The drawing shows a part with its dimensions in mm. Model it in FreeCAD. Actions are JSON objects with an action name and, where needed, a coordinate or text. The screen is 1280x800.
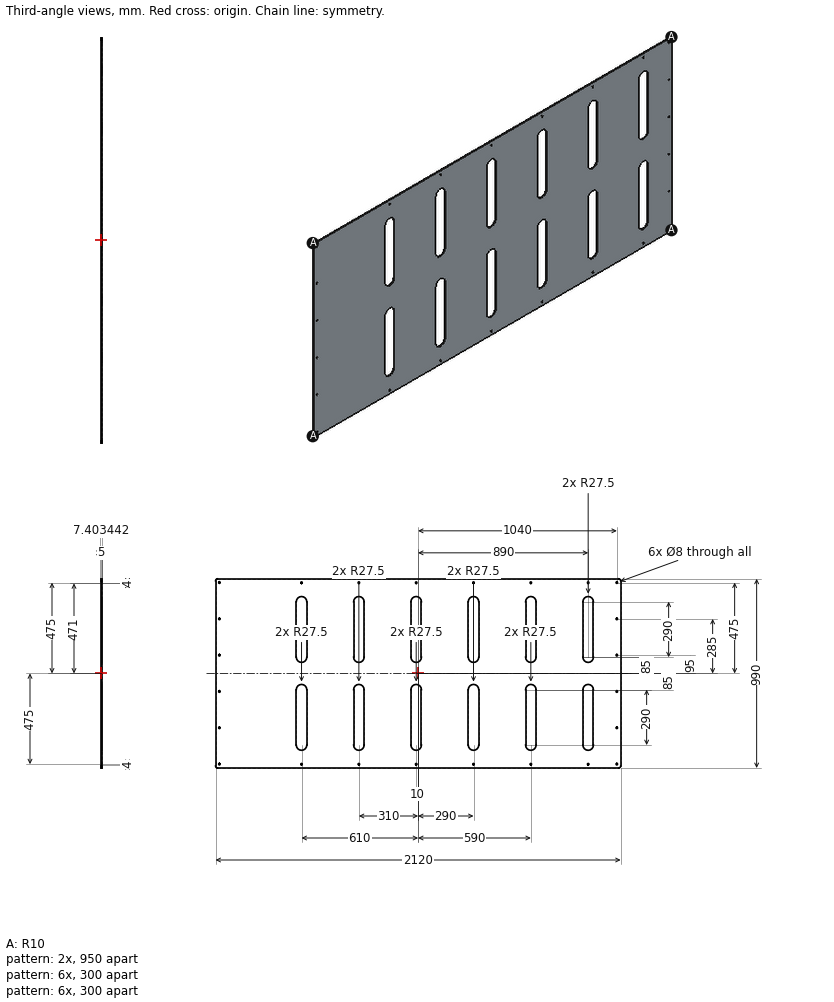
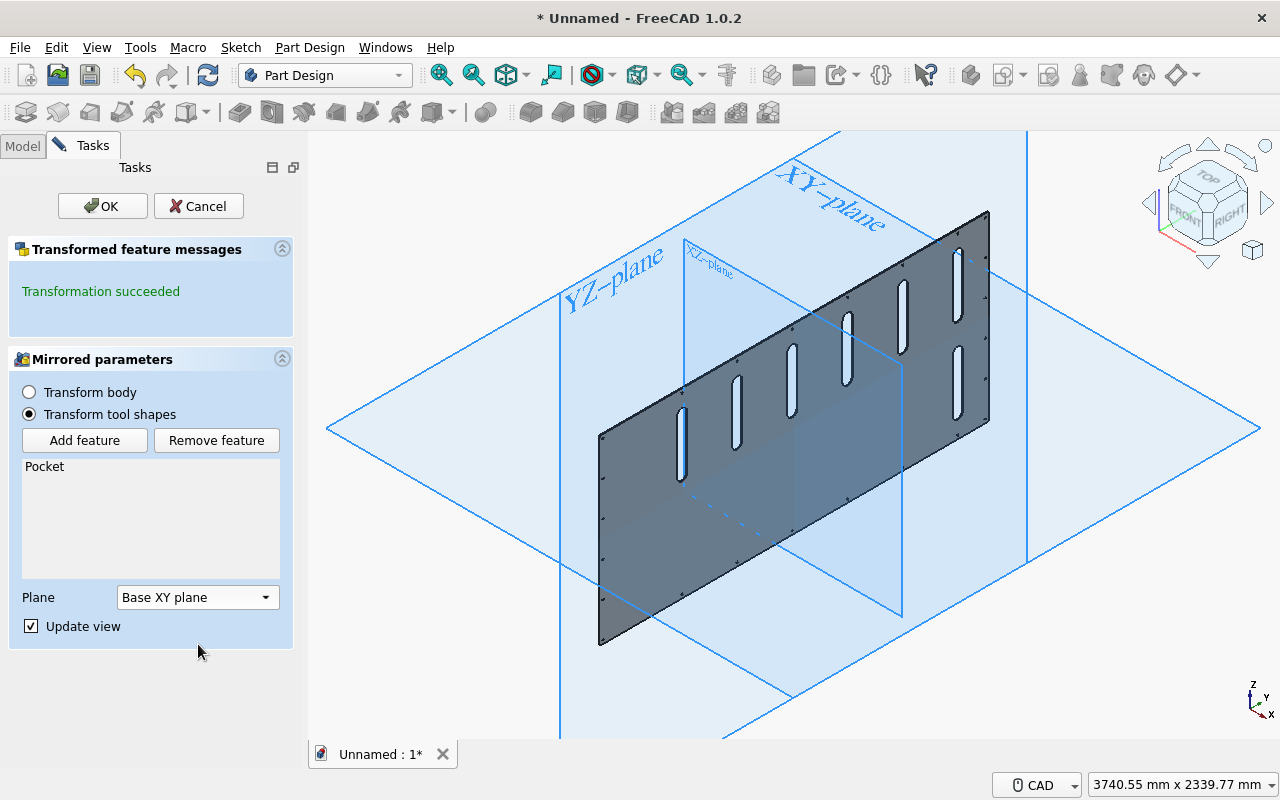
{"action": "left_click", "coordinate": [103, 206]}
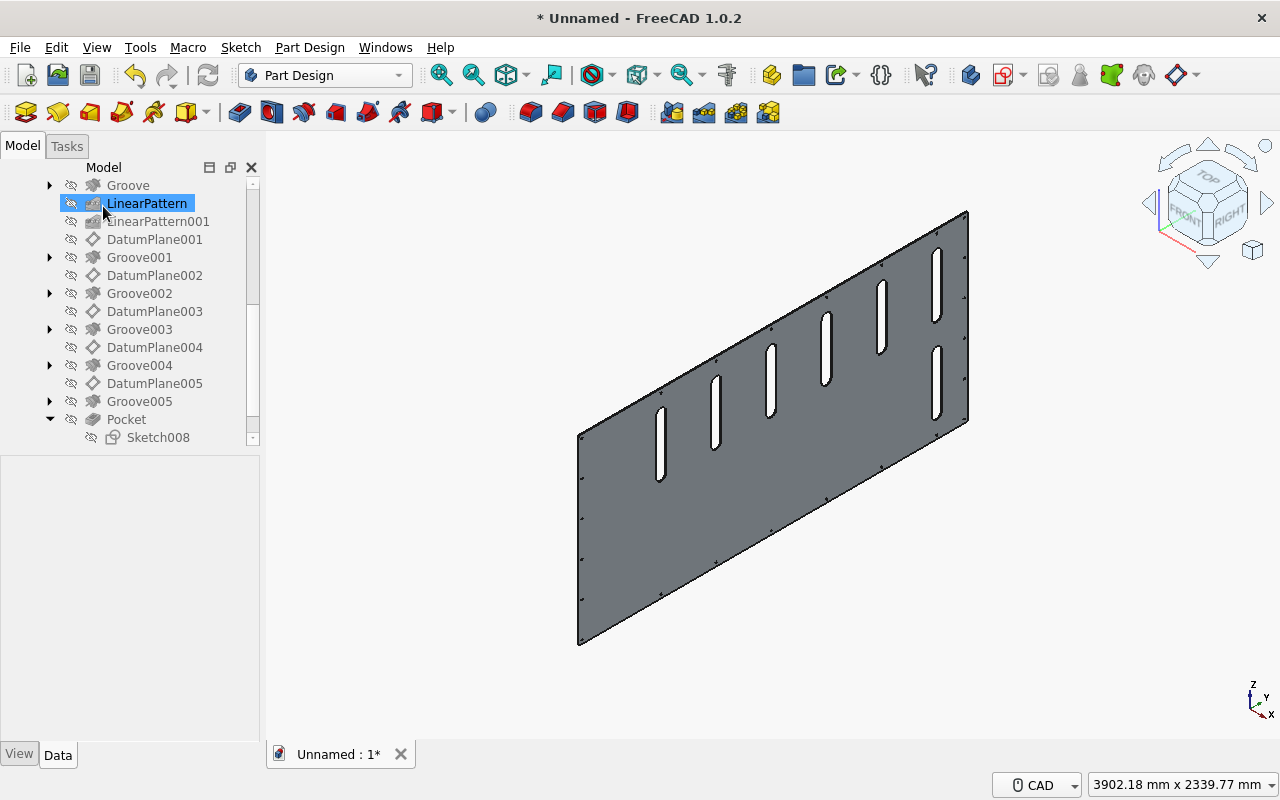
{"action": "left_click", "coordinate": [885, 393]}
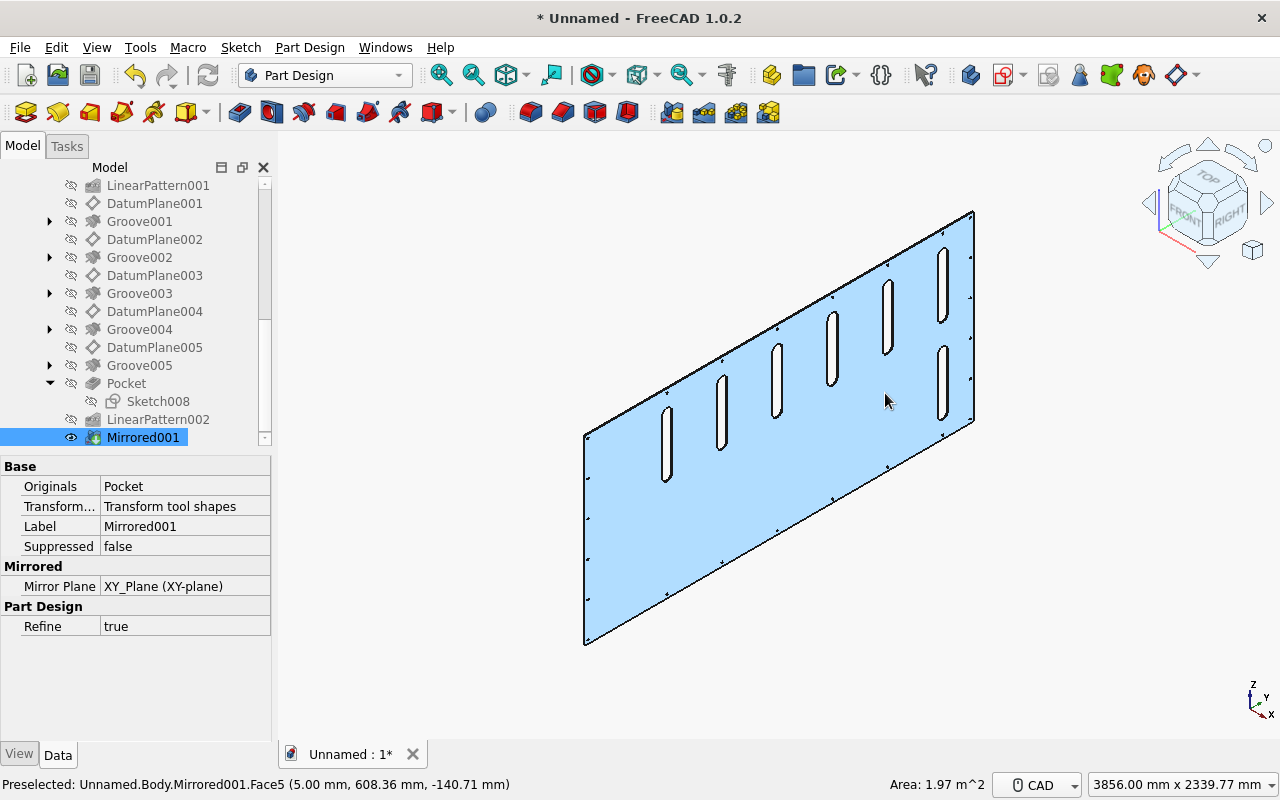
{"action": "left_click", "coordinate": [1004, 76]}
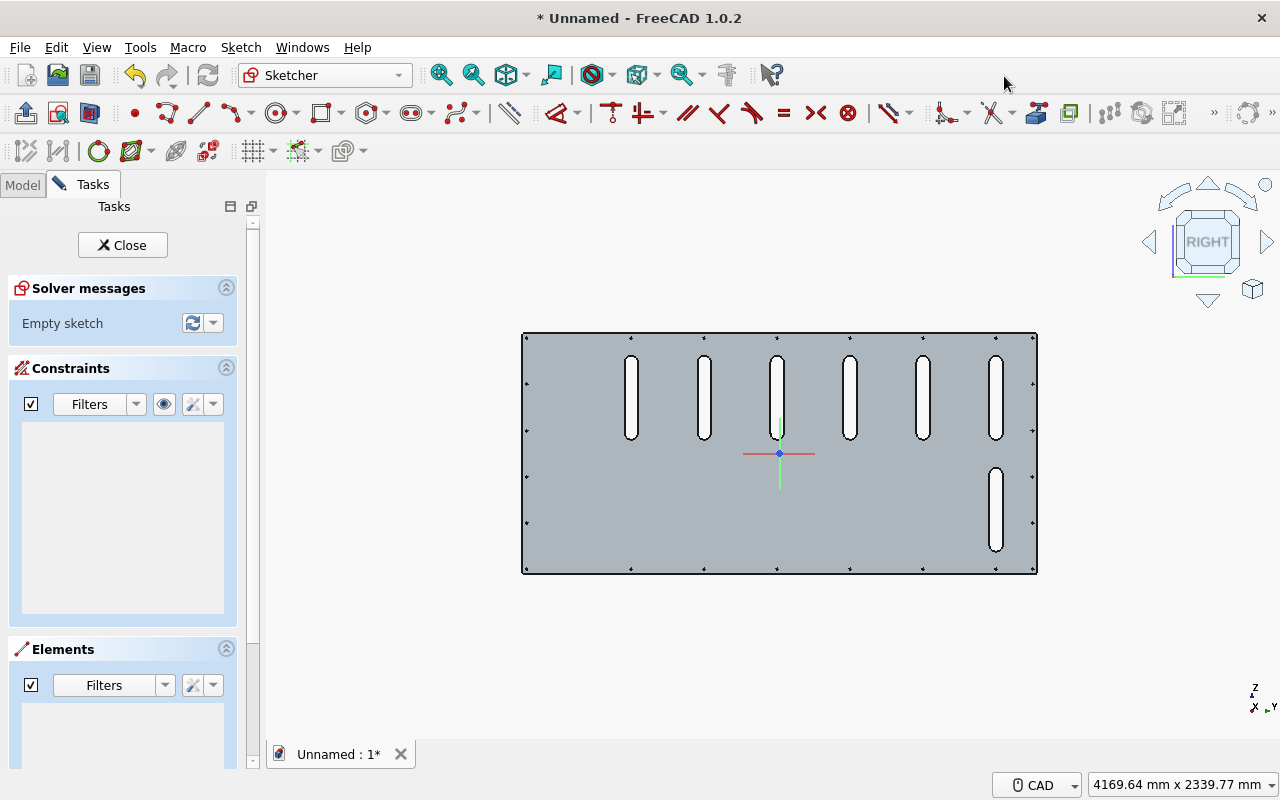
{"action": "scroll", "coordinate": [904, 518], "scroll_direction": "up", "scroll_amount": 7}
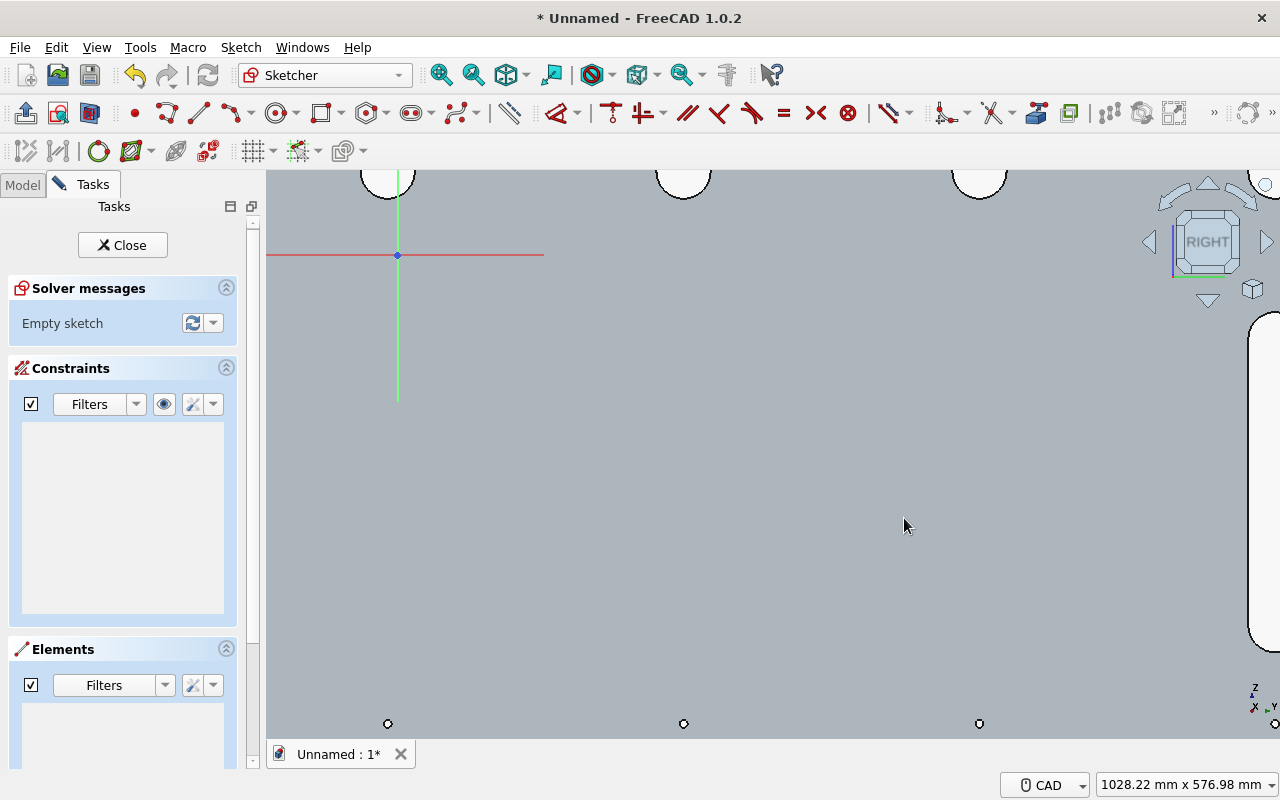
{"action": "left_click", "coordinate": [412, 114]}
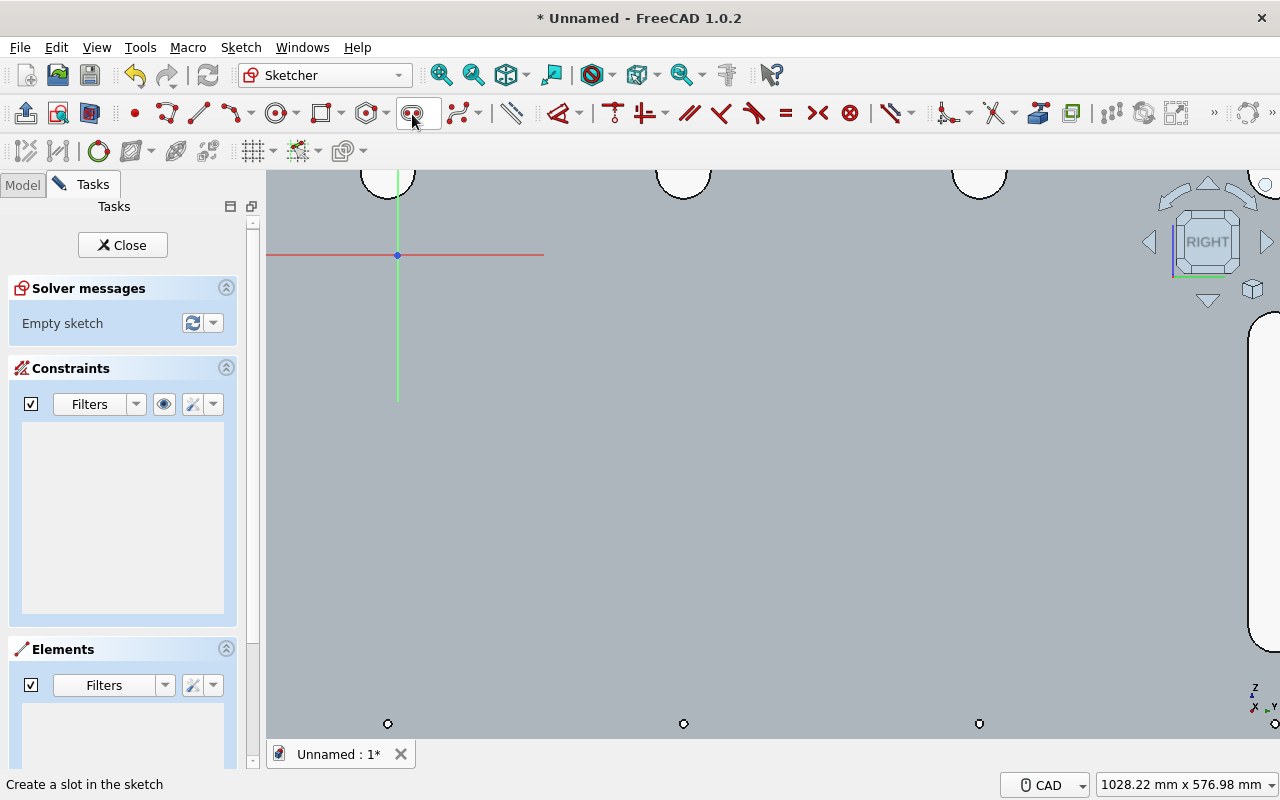
{"action": "left_click", "coordinate": [979, 625]}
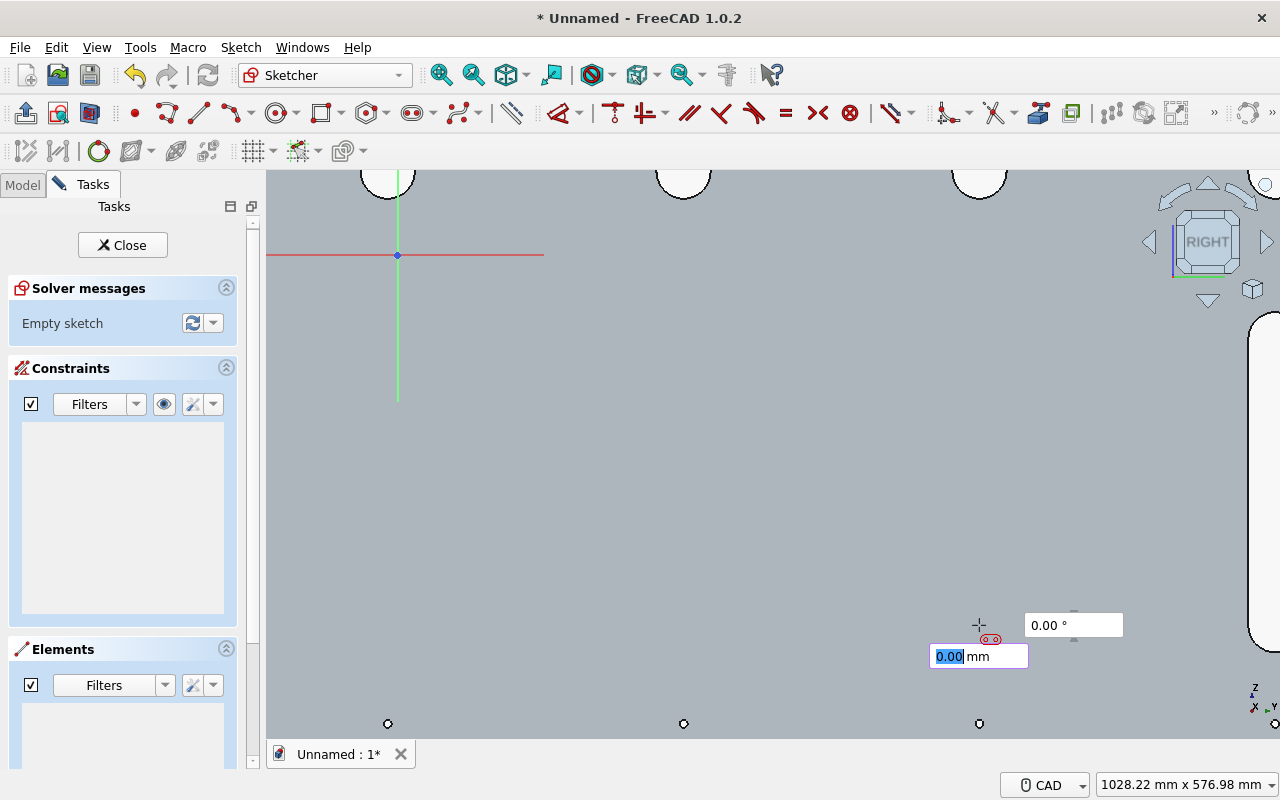
{"action": "left_click", "coordinate": [979, 339]}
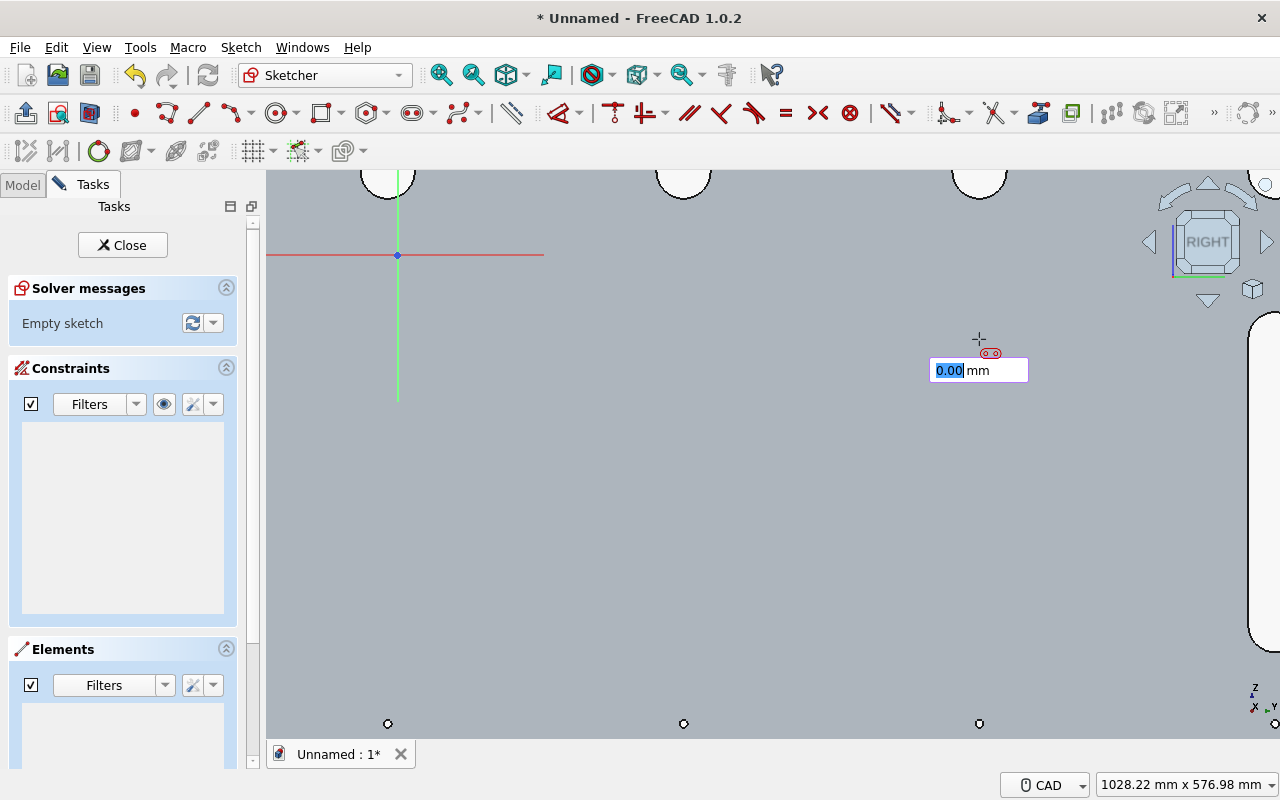
{"action": "left_click", "coordinate": [1007, 482]}
{"action": "key", "text": "Escape"}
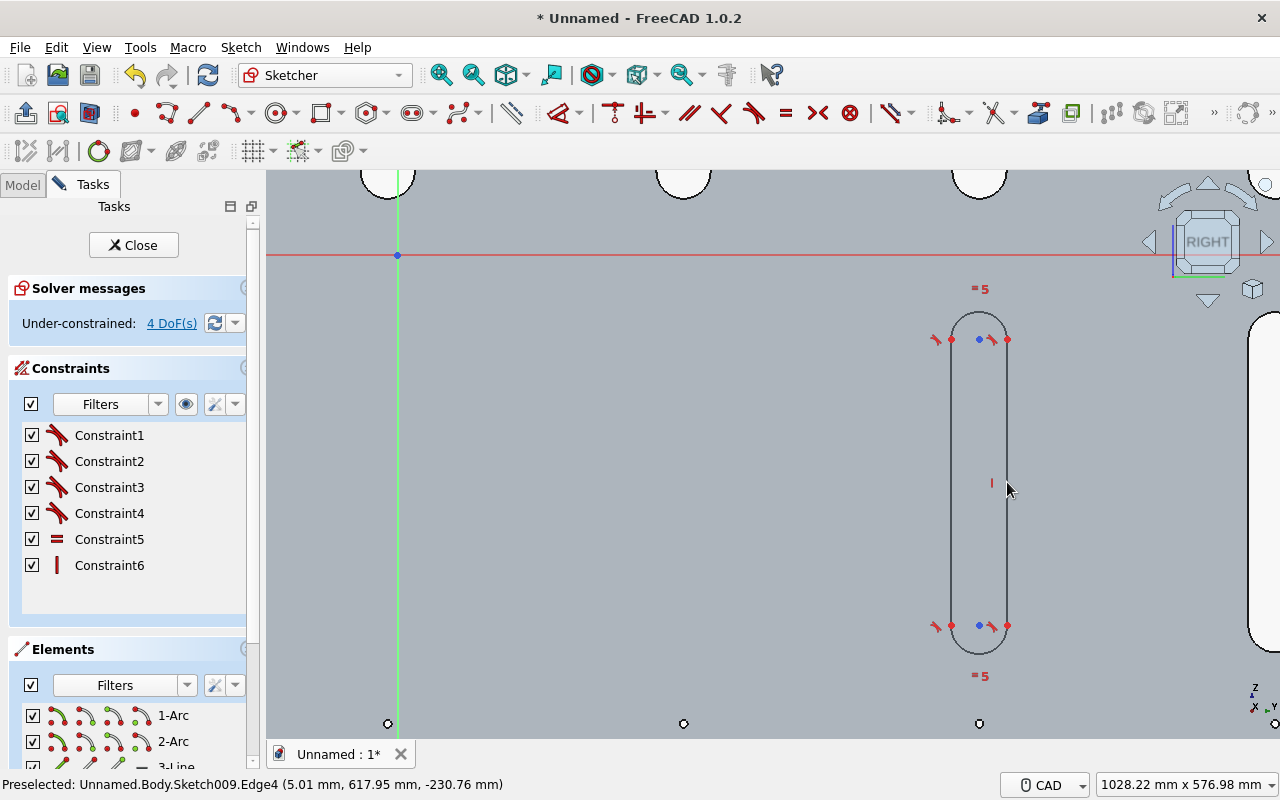
{"action": "left_click", "coordinate": [558, 114]}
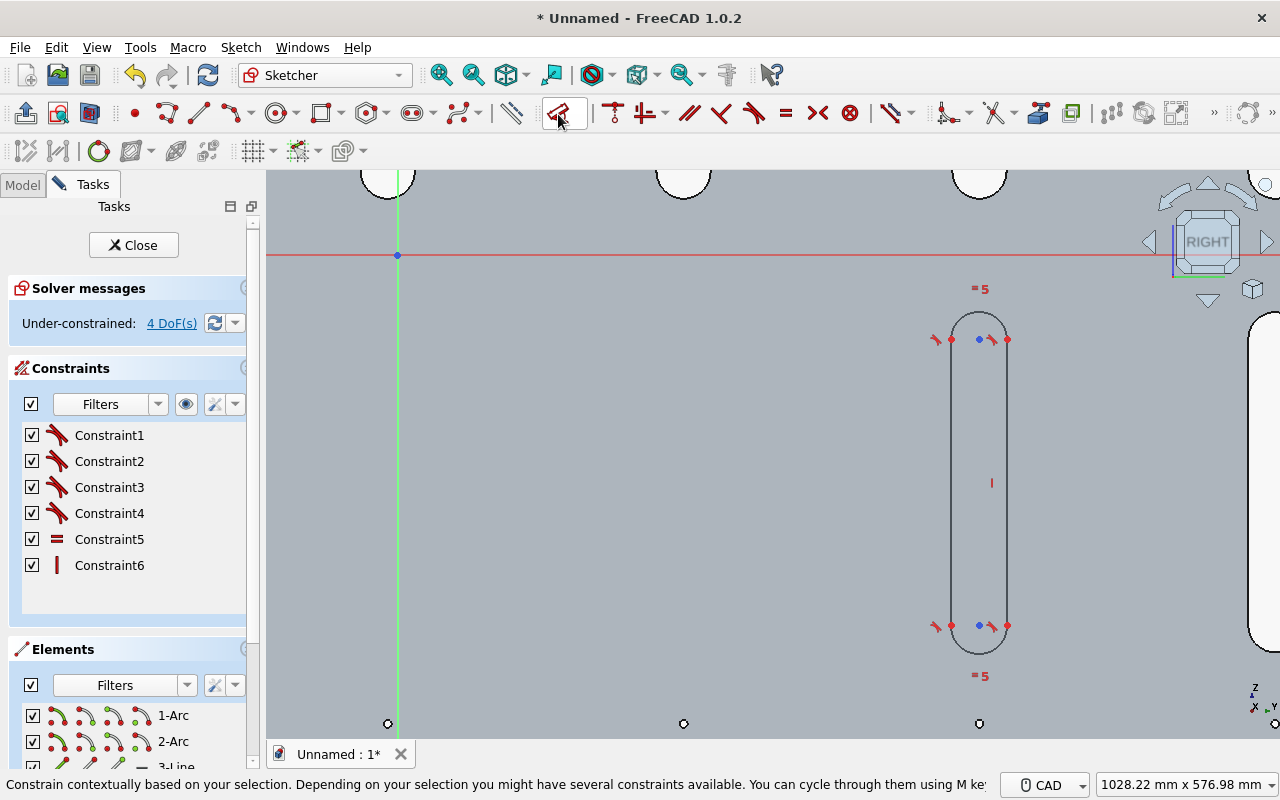
{"action": "scroll", "coordinate": [963, 649], "scroll_direction": "up", "scroll_amount": 2}